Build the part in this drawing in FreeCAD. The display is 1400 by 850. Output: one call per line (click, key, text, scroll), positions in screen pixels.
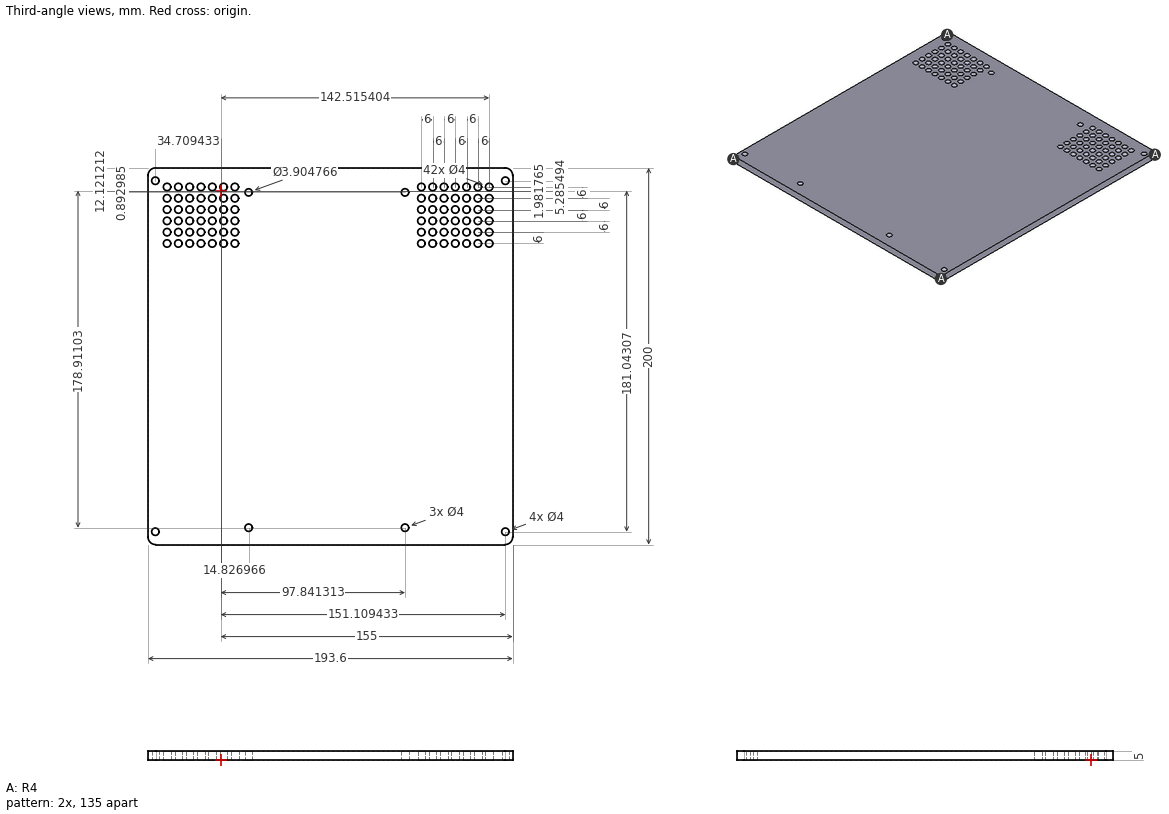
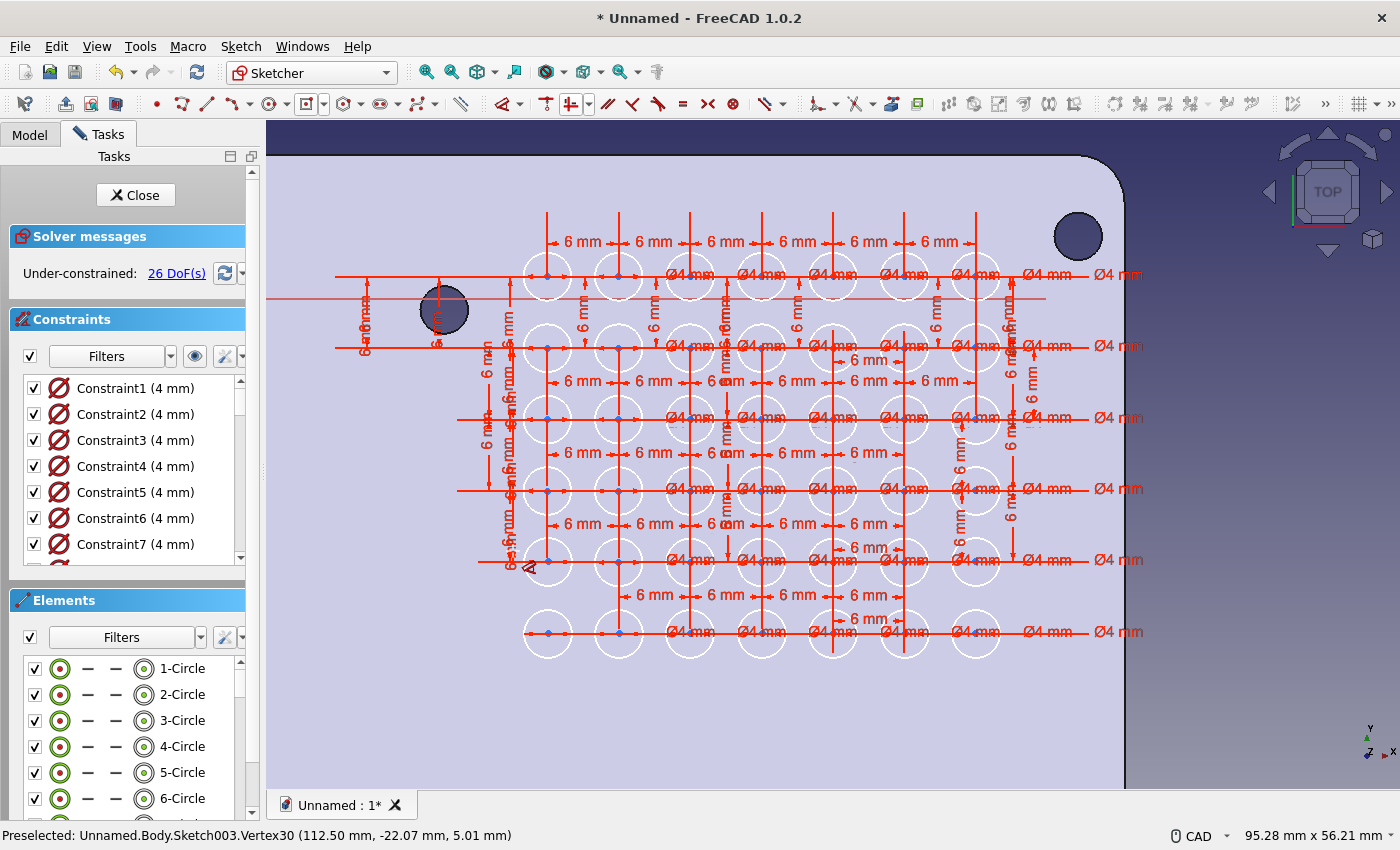
click(619, 562)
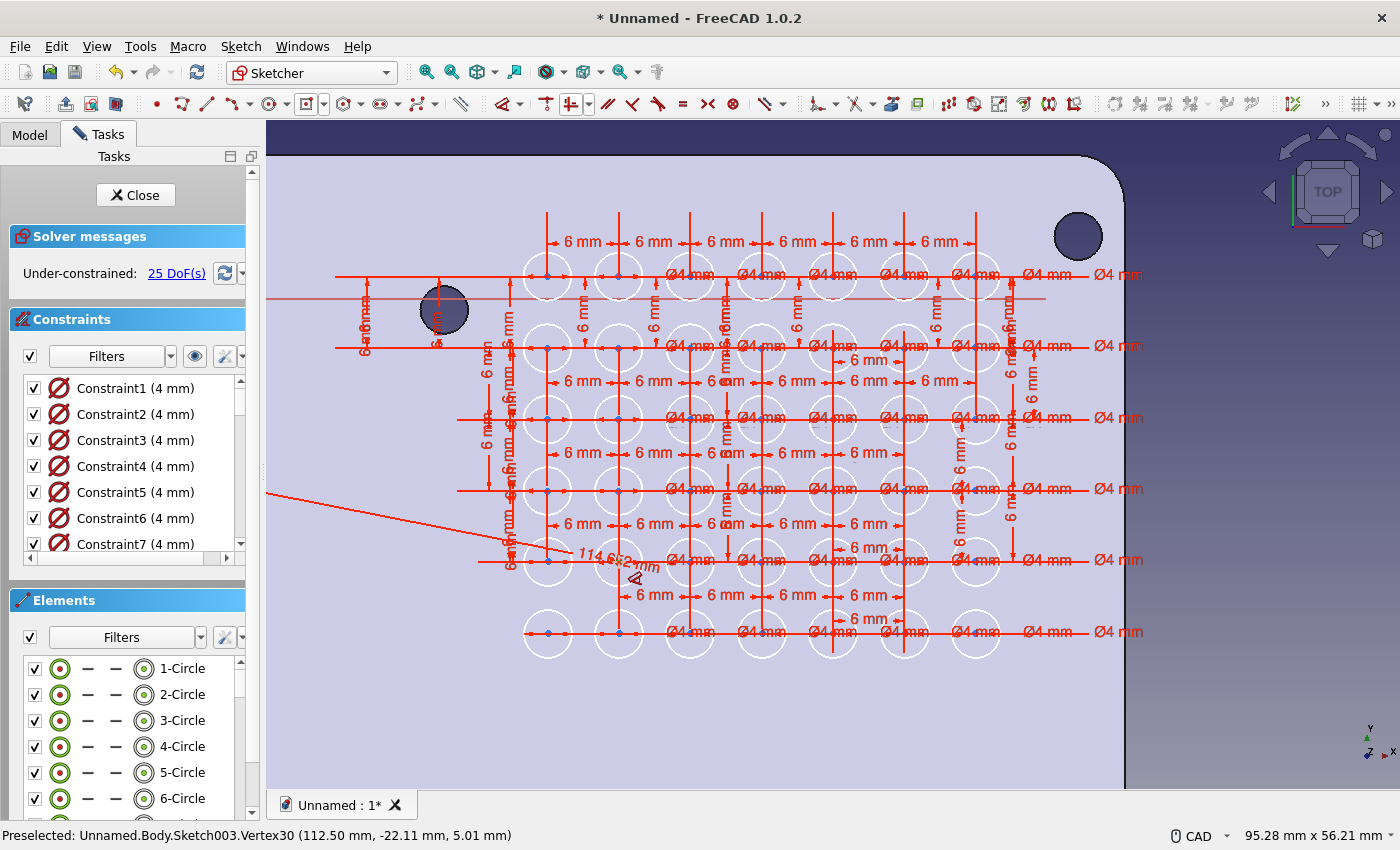
click(548, 562)
click(583, 596)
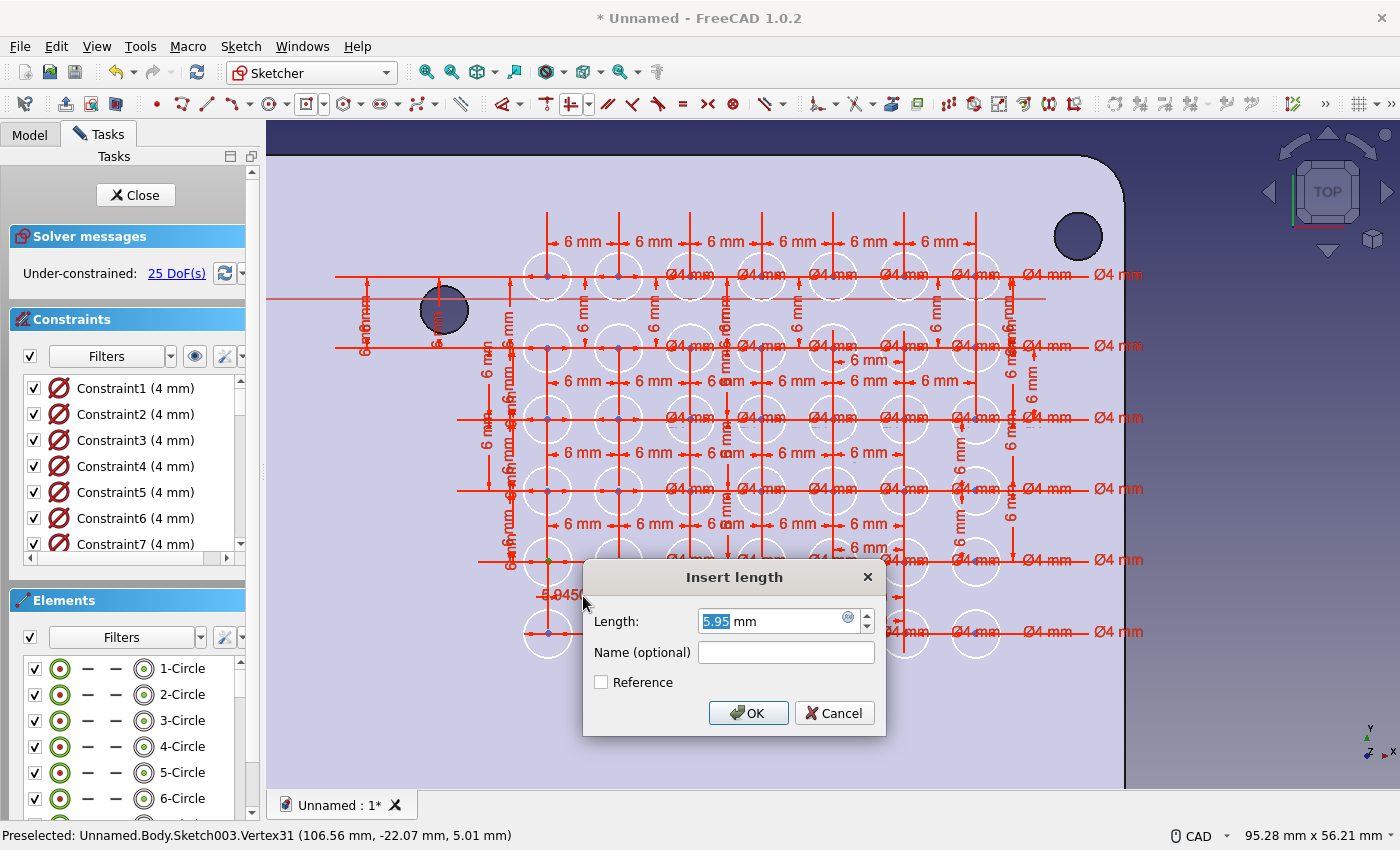
text(6)
key(Return)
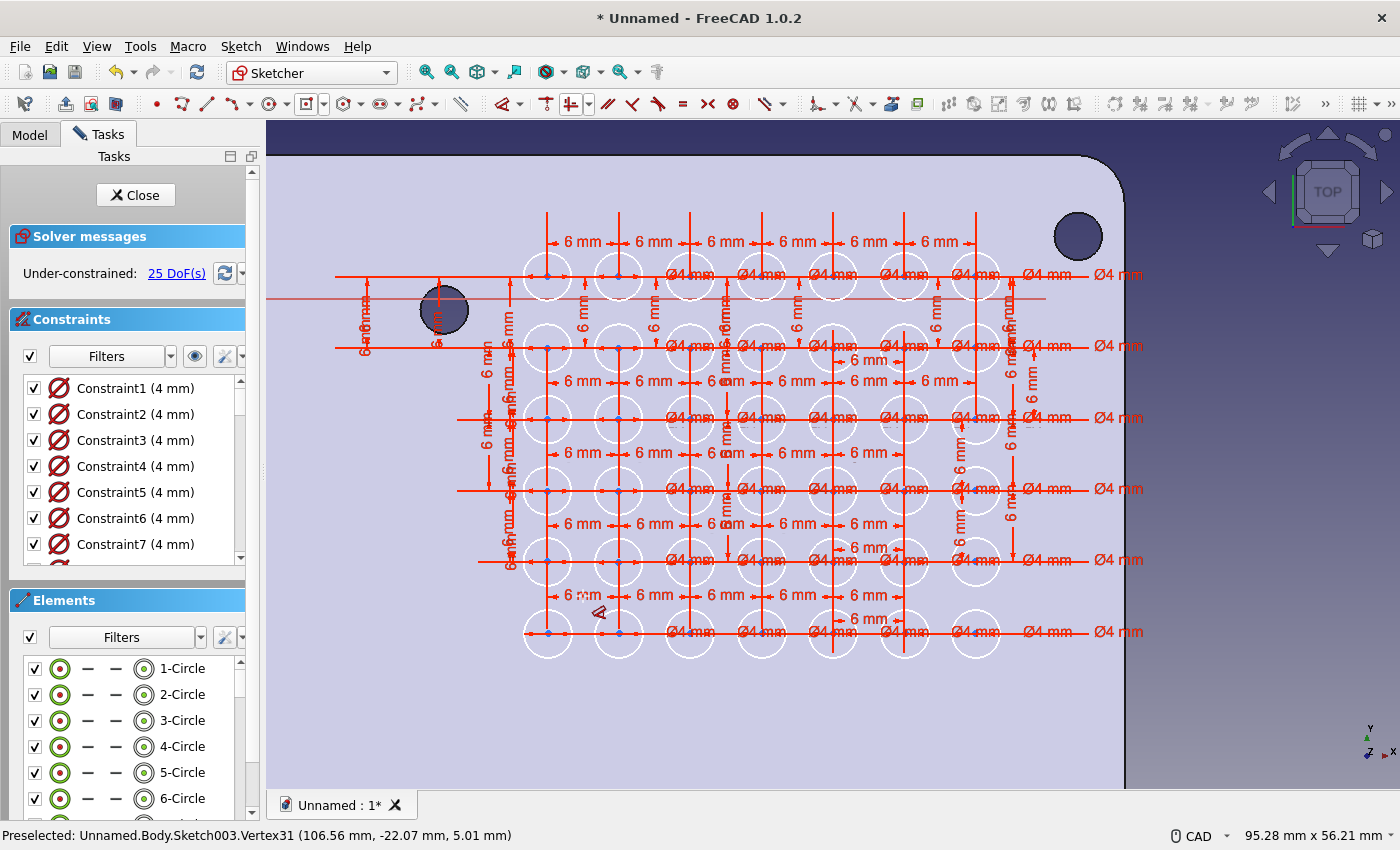
click(547, 491)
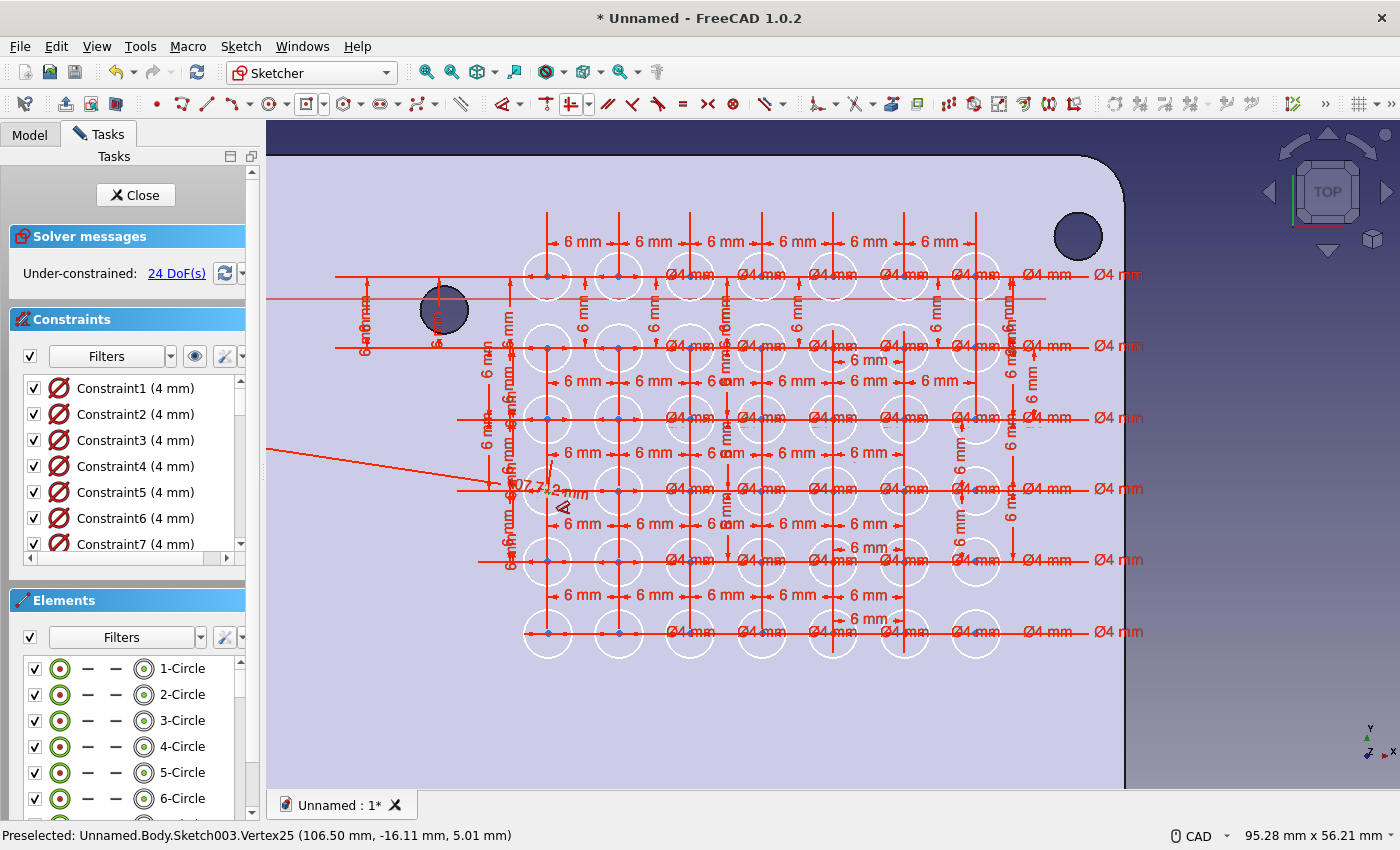
click(547, 562)
click(489, 502)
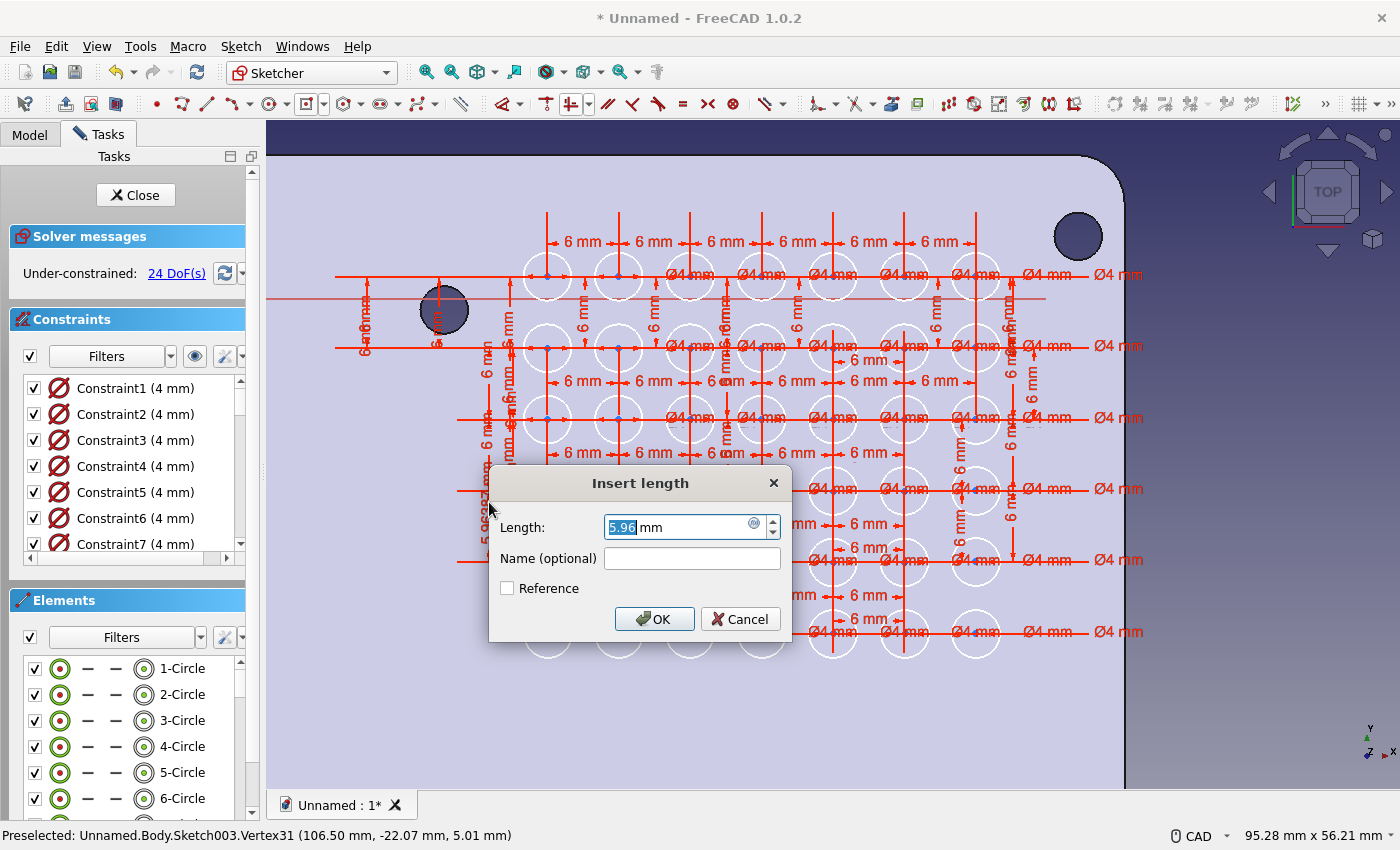
text(6)
key(Return)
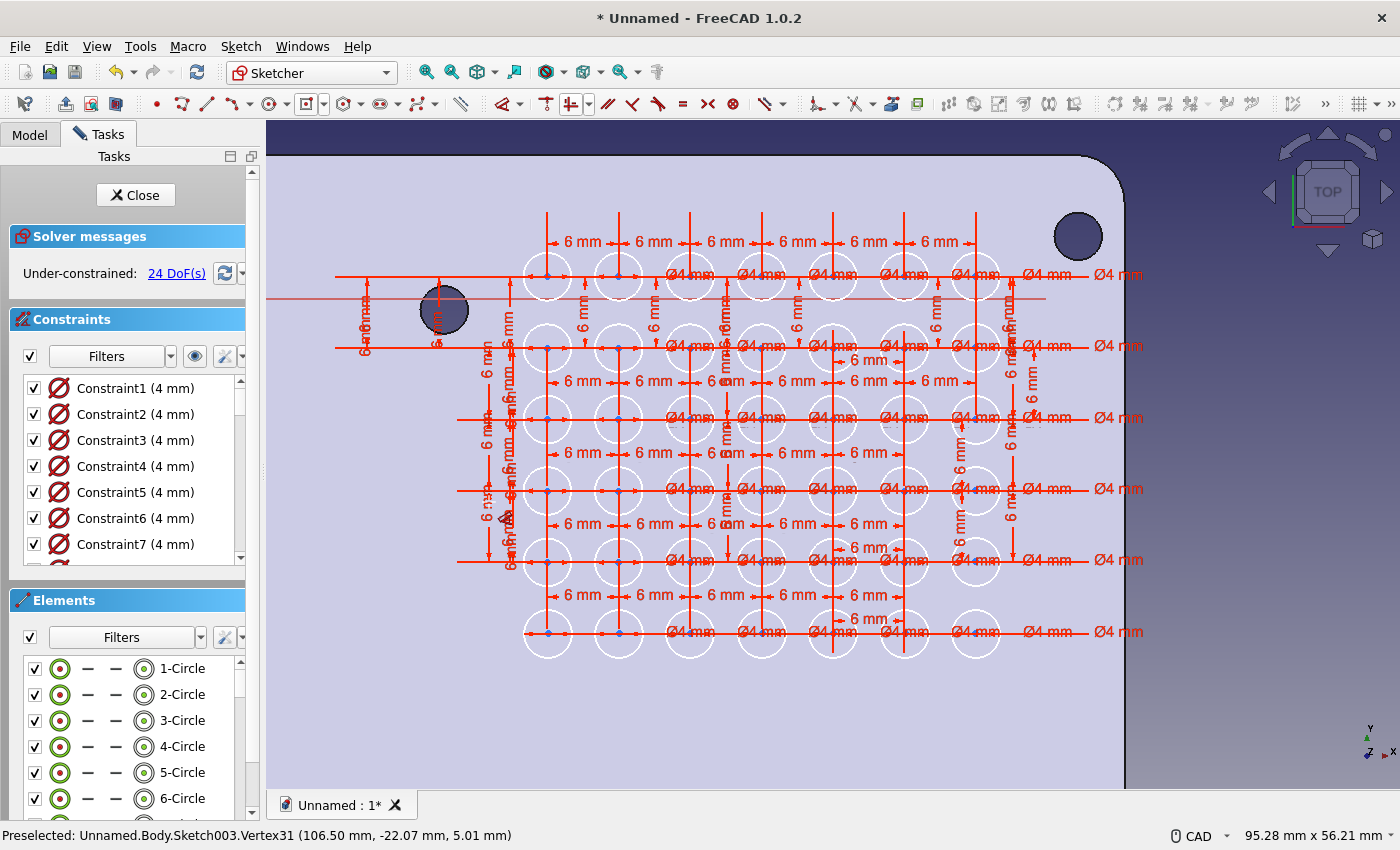
click(833, 562)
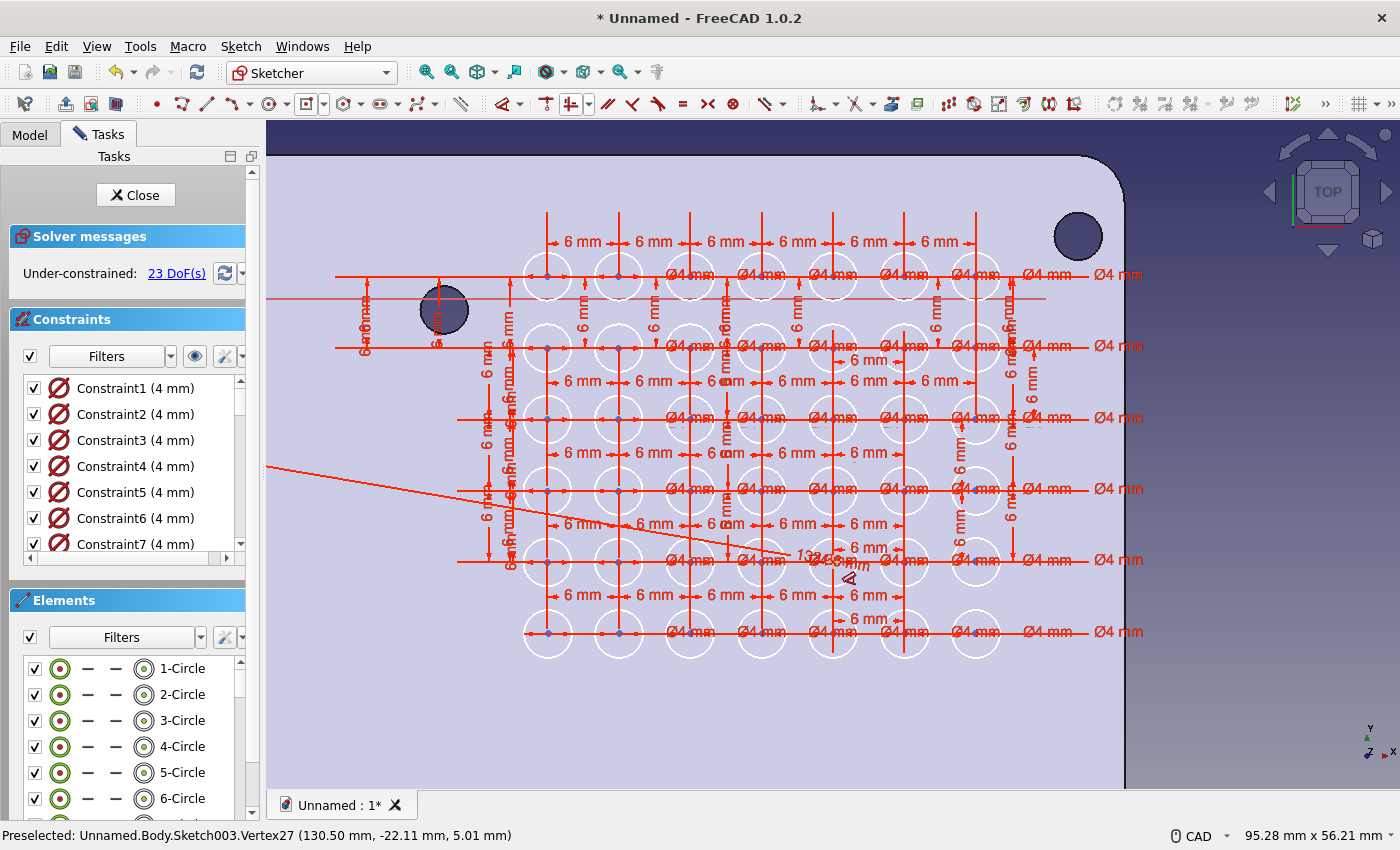
click(905, 634)
click(869, 668)